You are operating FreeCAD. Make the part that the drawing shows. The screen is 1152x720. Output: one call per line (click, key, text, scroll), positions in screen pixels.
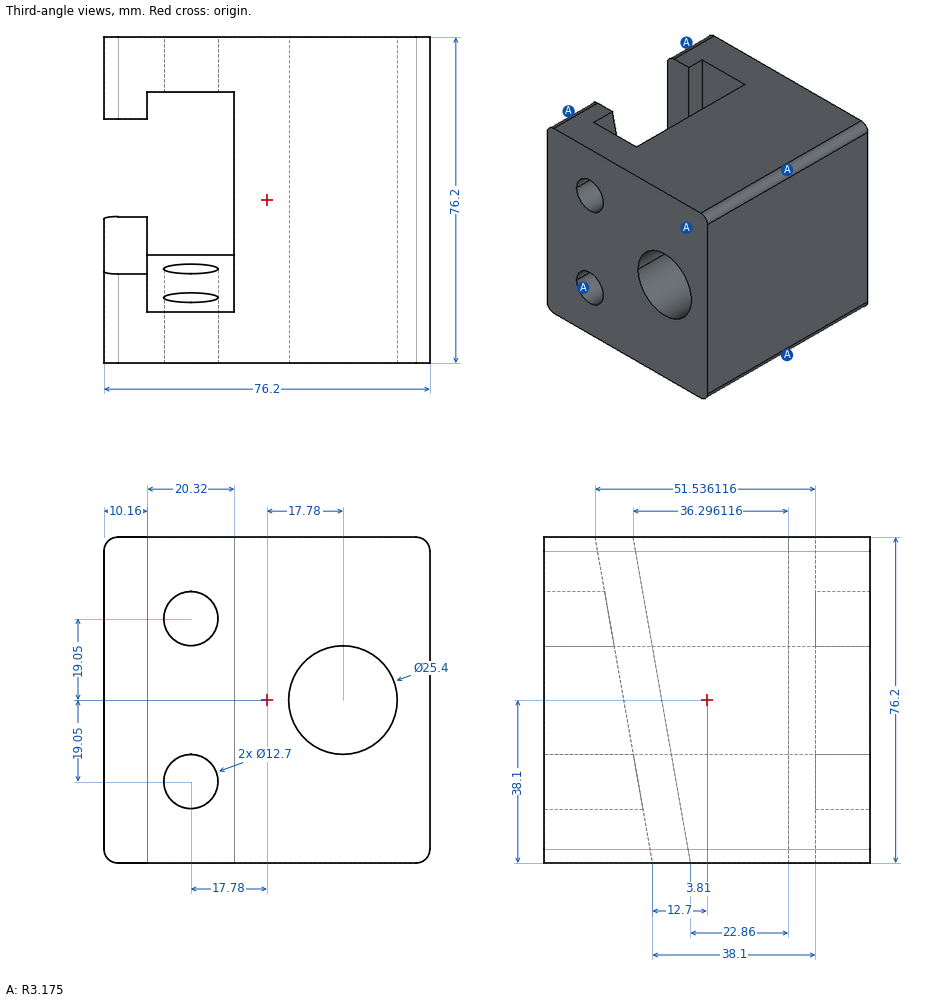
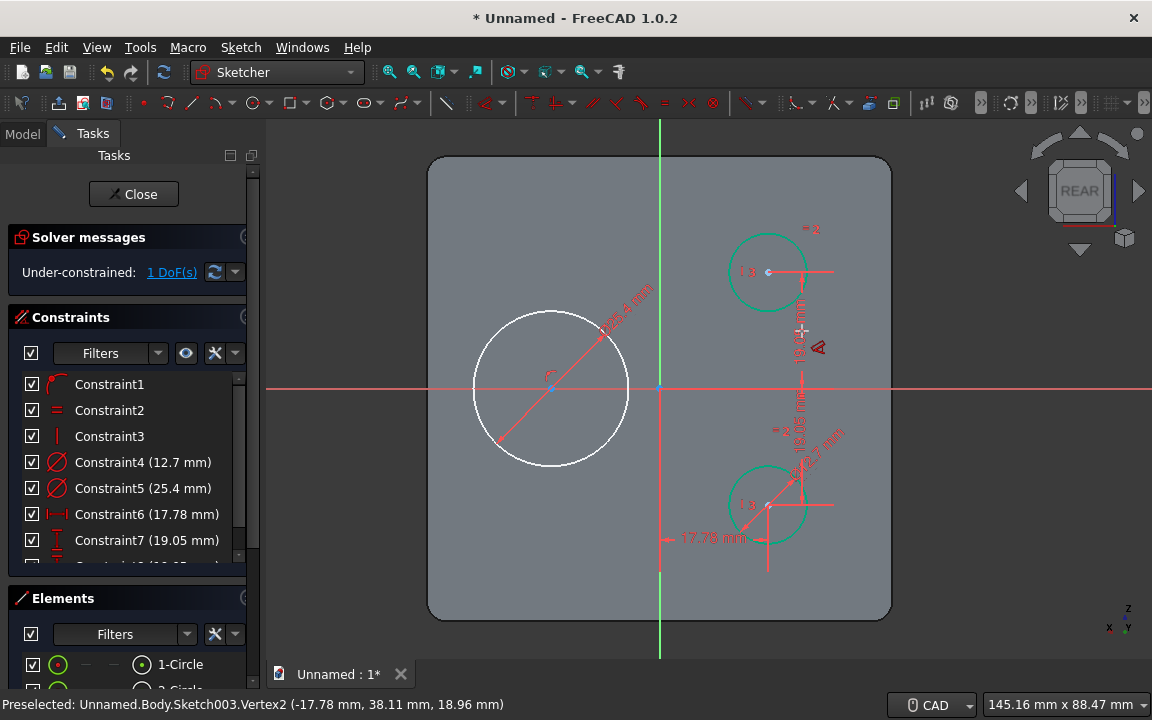
click(551, 389)
click(605, 423)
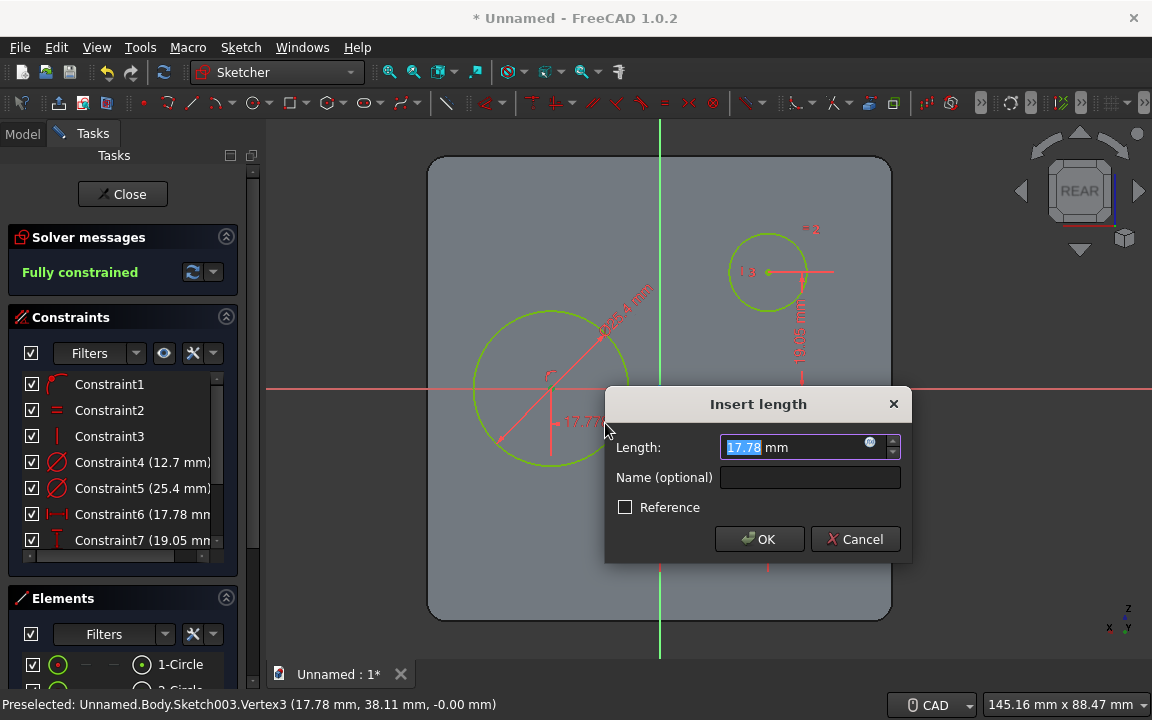
text(17.78)
key(Return)
key(Escape)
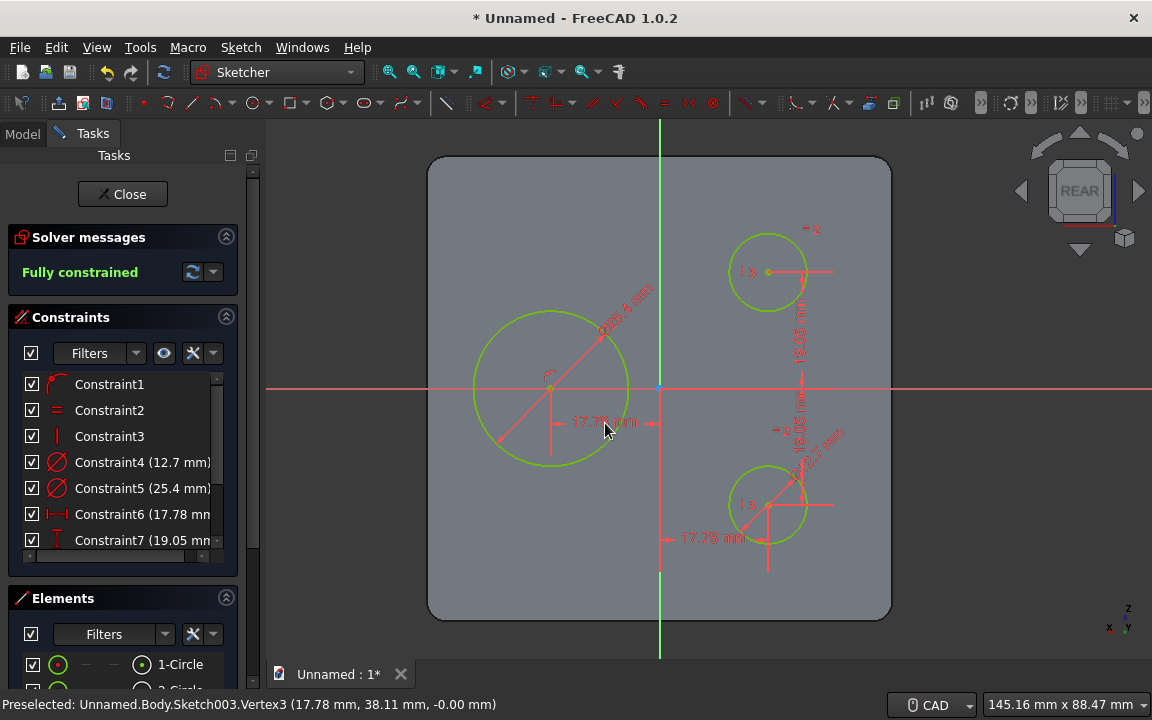
click(123, 194)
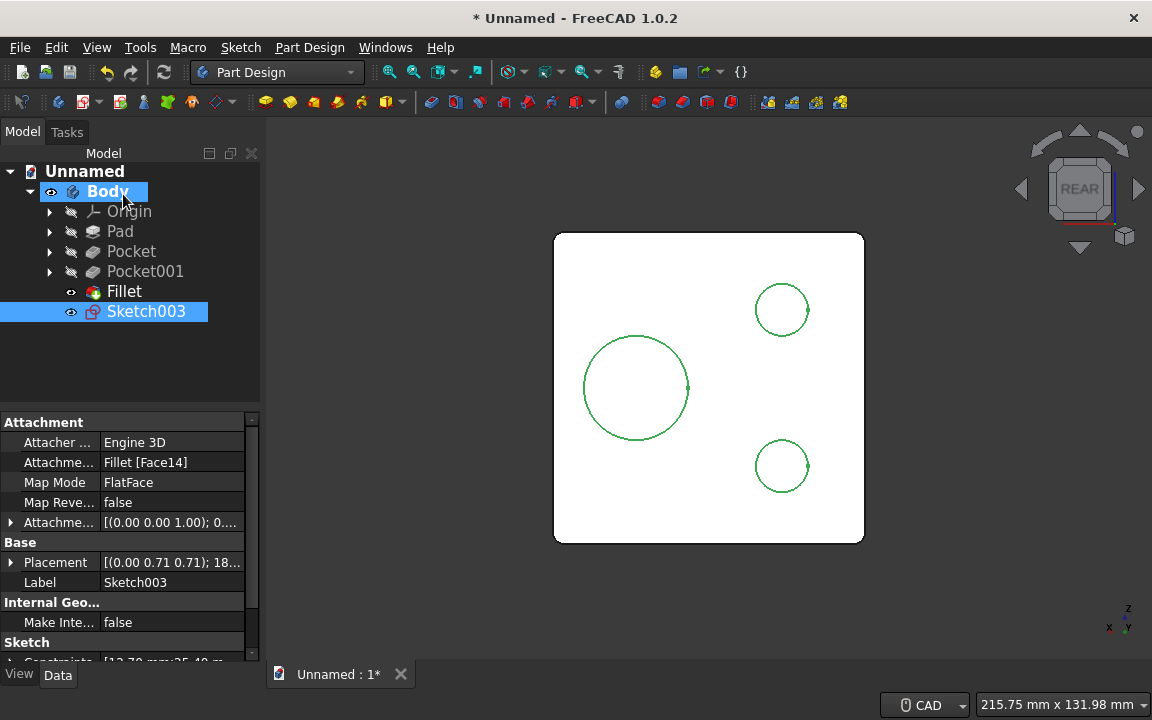
click(432, 102)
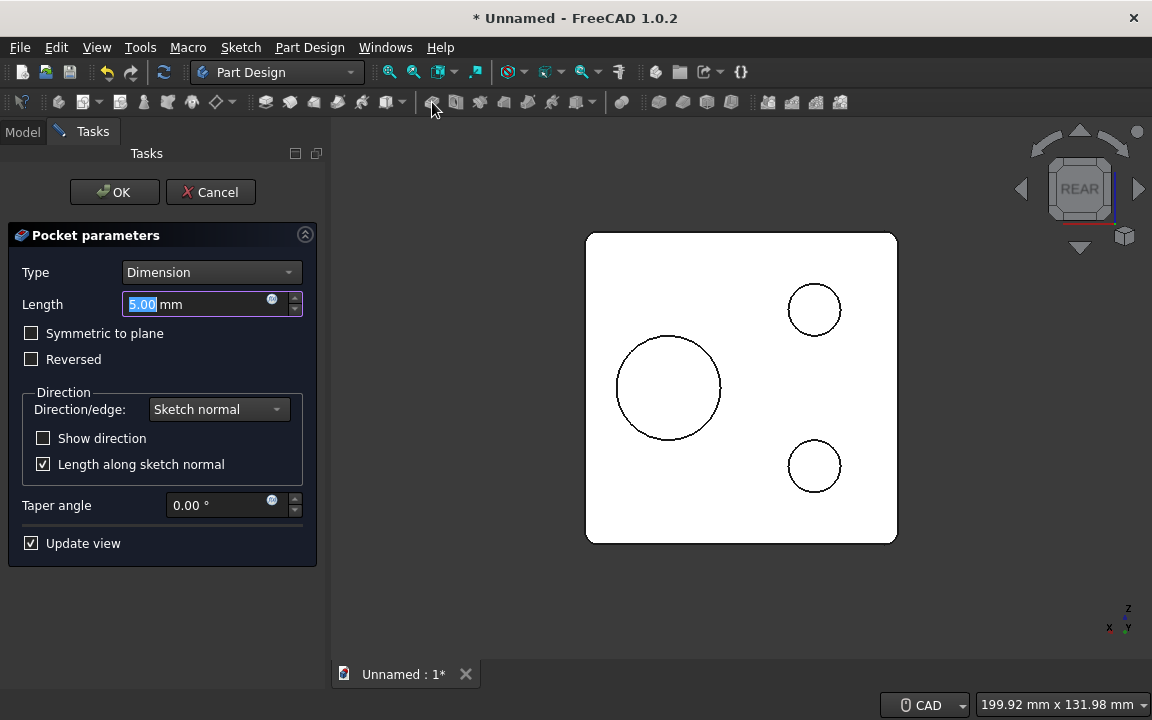
click(212, 272)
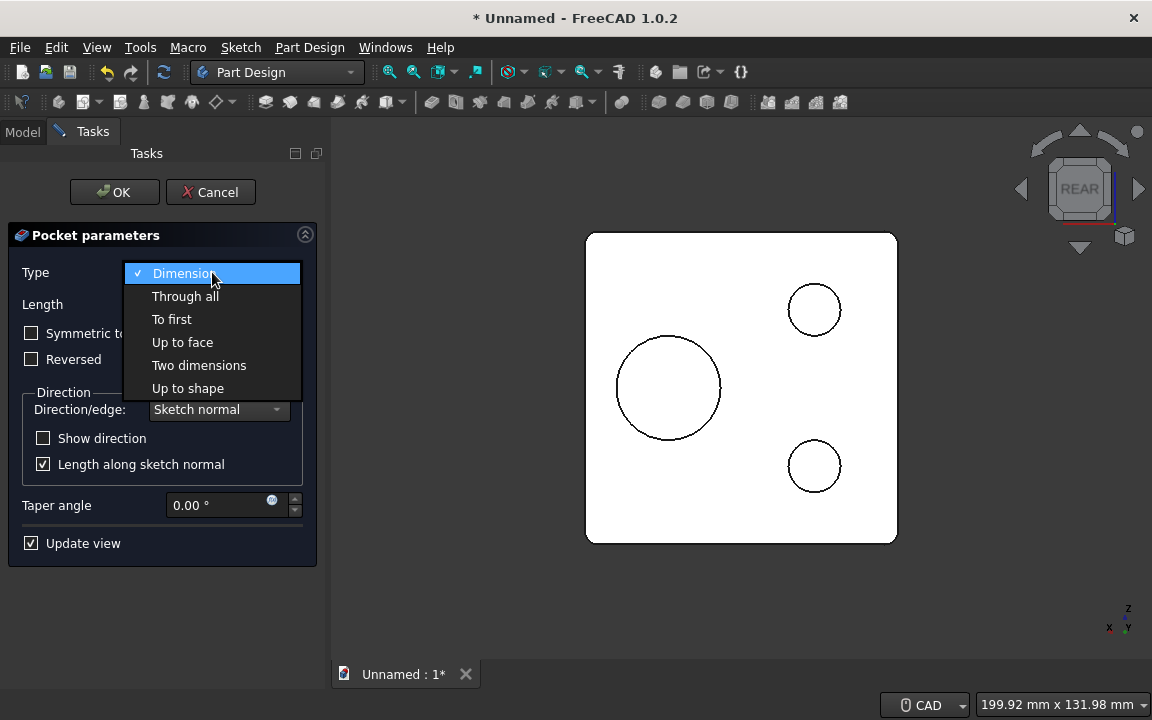
click(212, 296)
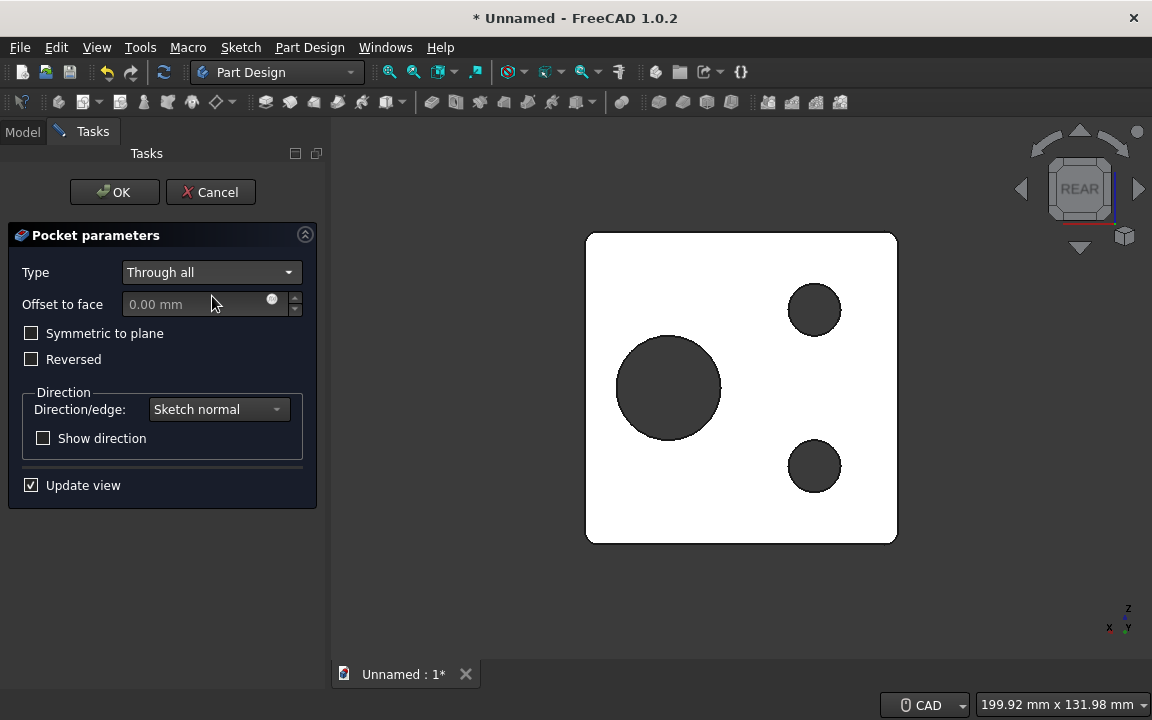
click(115, 192)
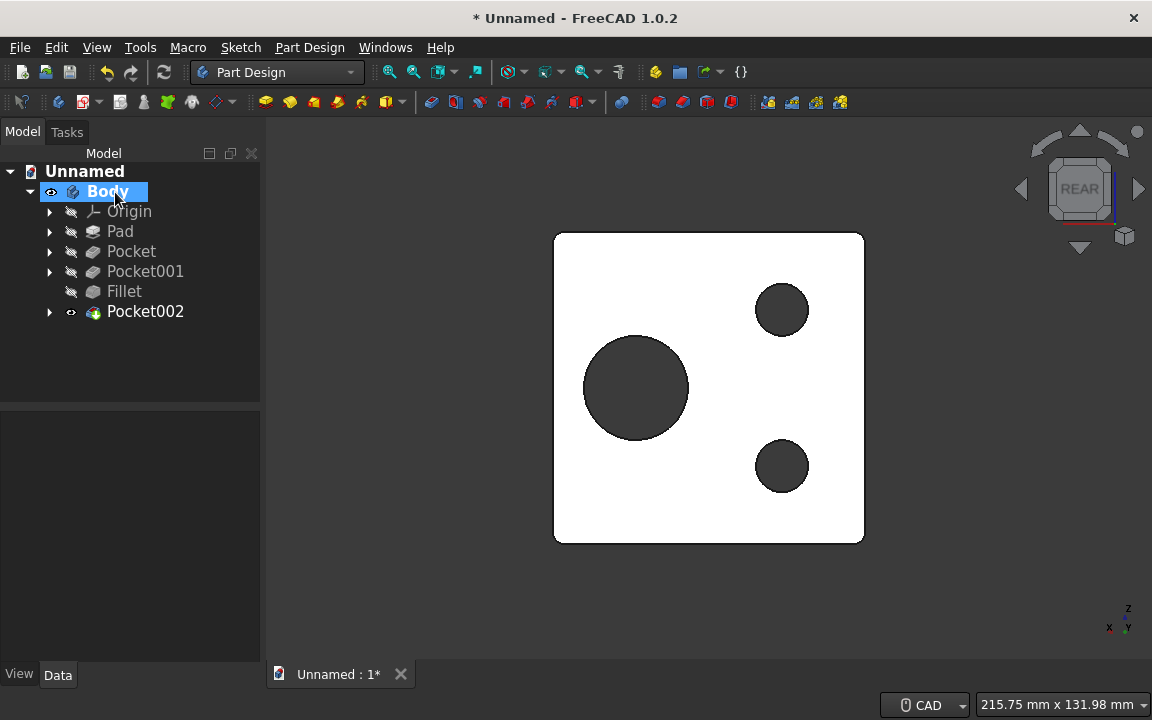
key(0)